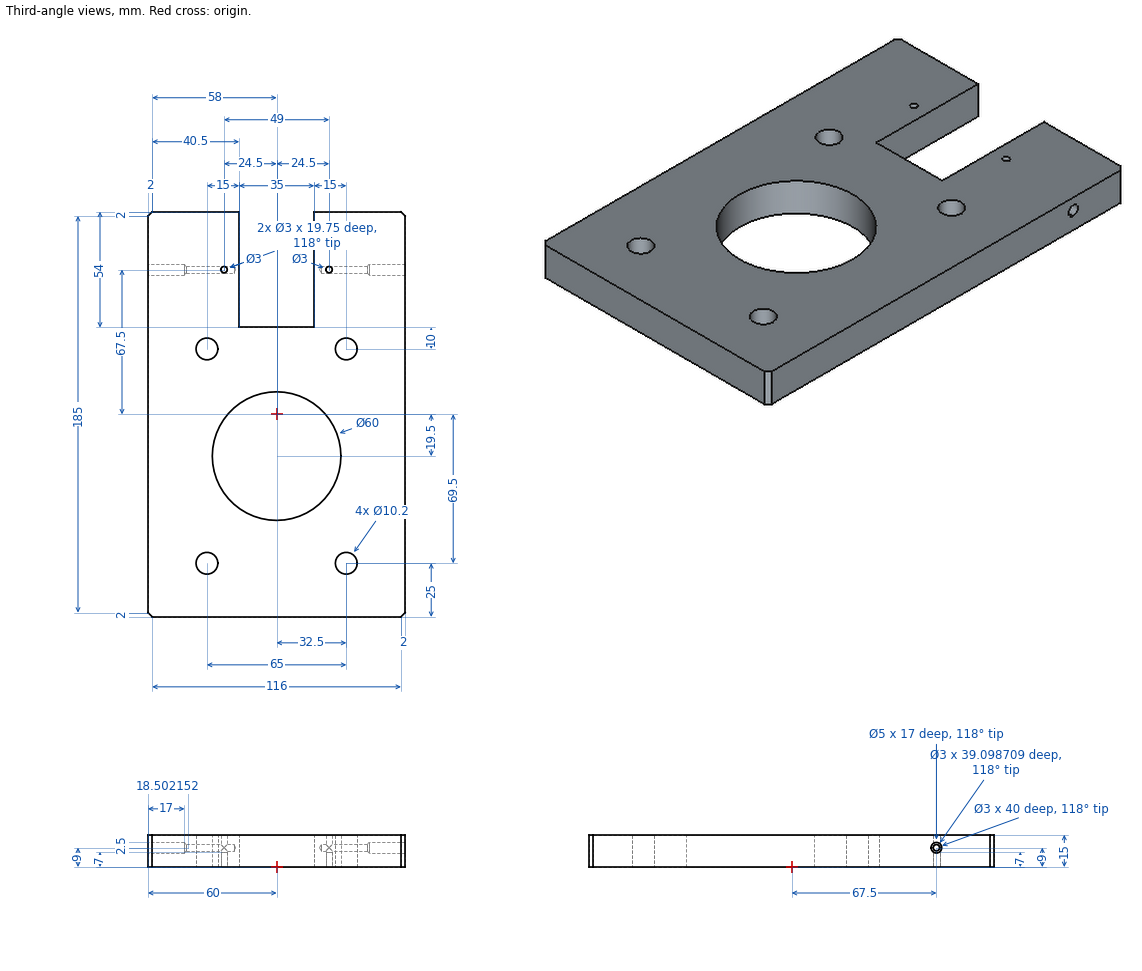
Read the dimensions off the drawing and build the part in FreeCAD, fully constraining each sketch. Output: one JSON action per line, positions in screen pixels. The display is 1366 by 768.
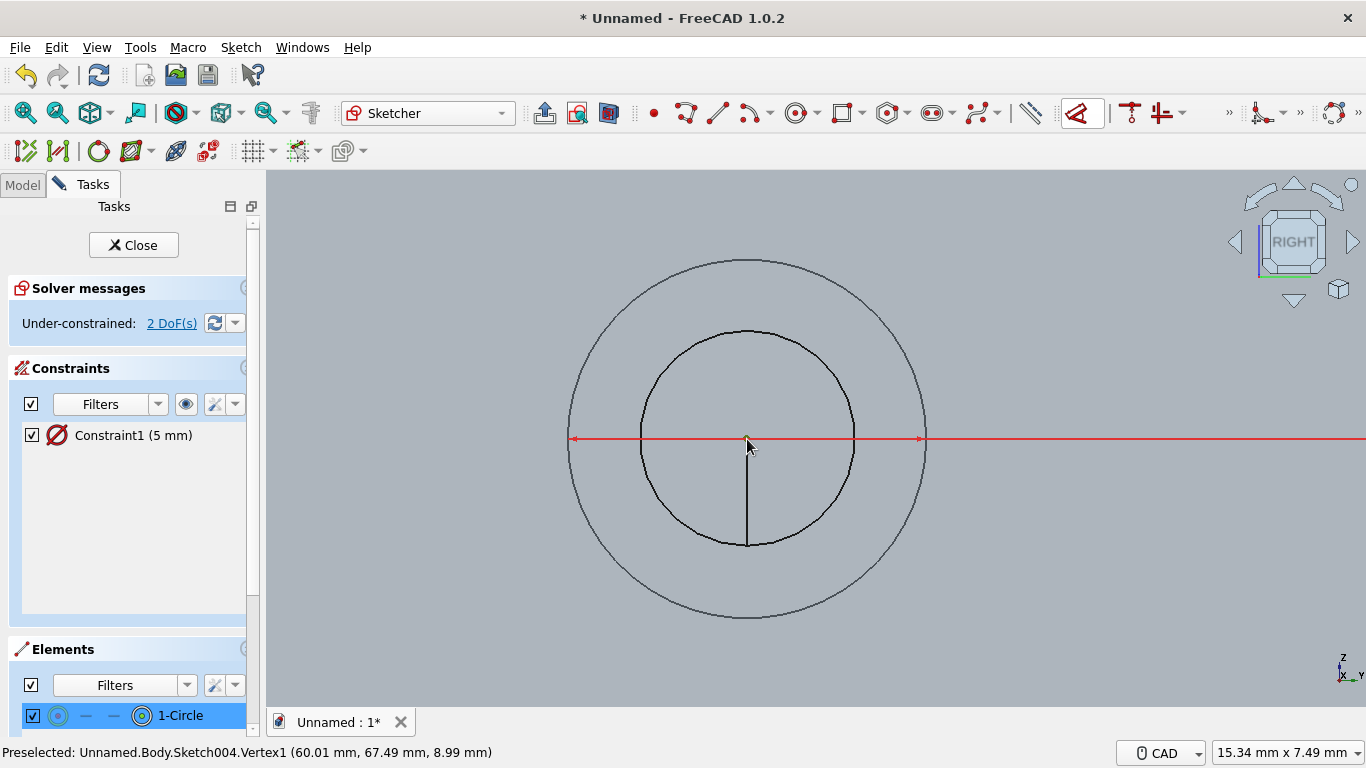
{"action": "key", "text": "i"}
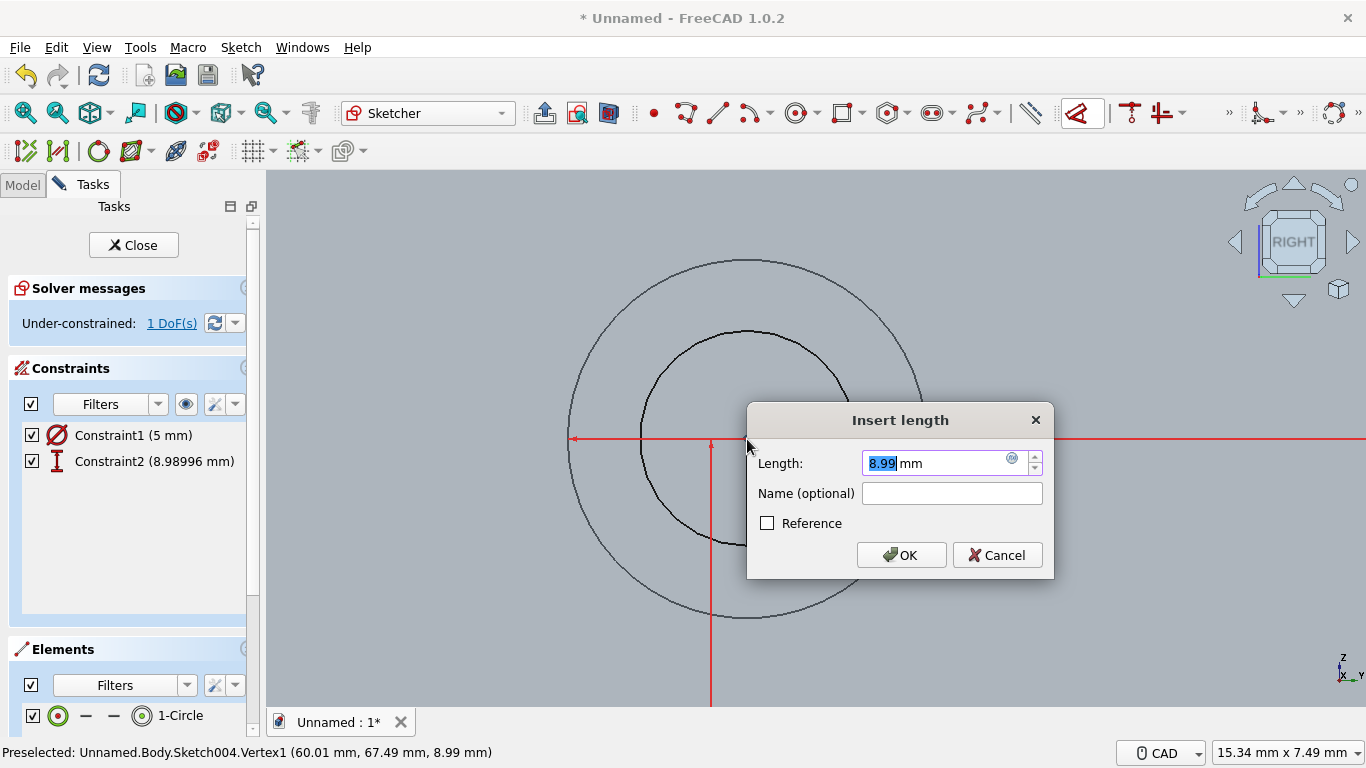
{"action": "type", "text": "9"}
{"action": "key", "text": "Return"}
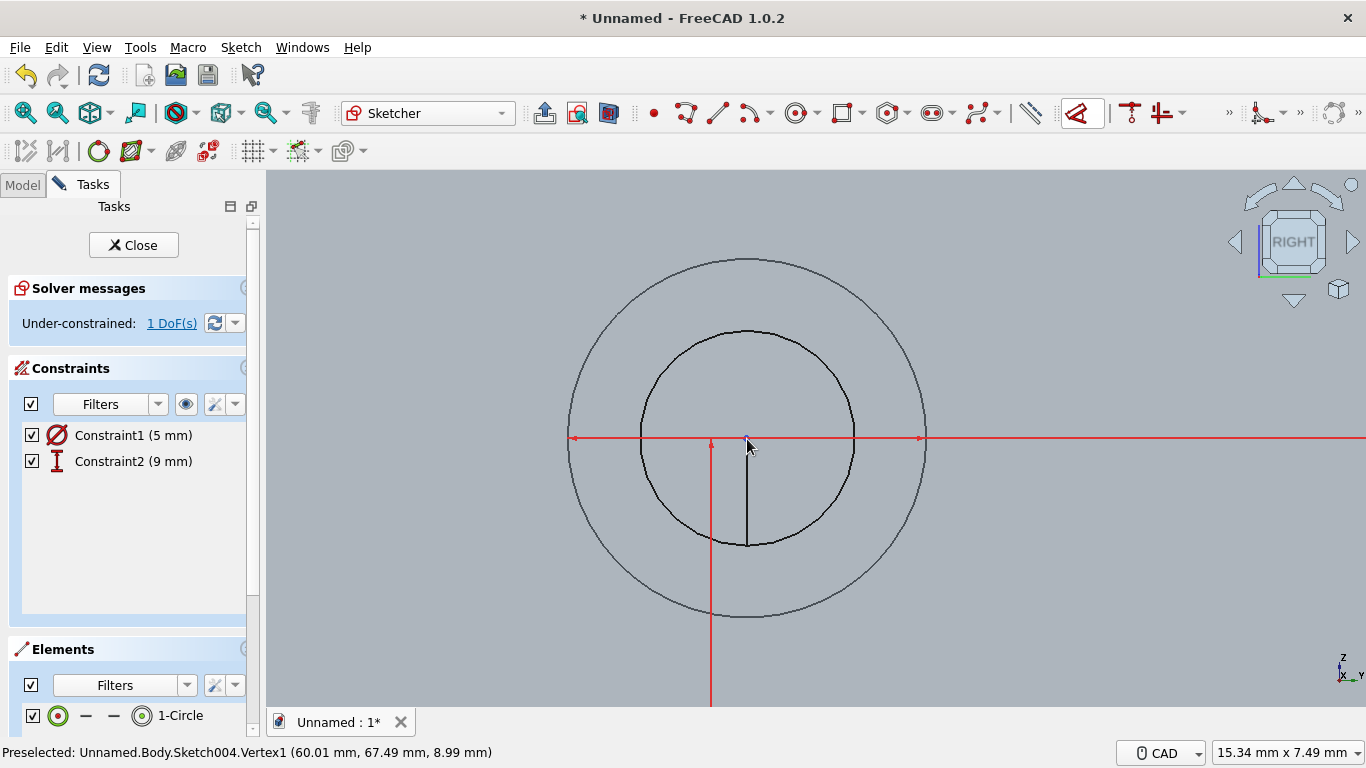
{"action": "left_click", "coordinate": [747, 438]}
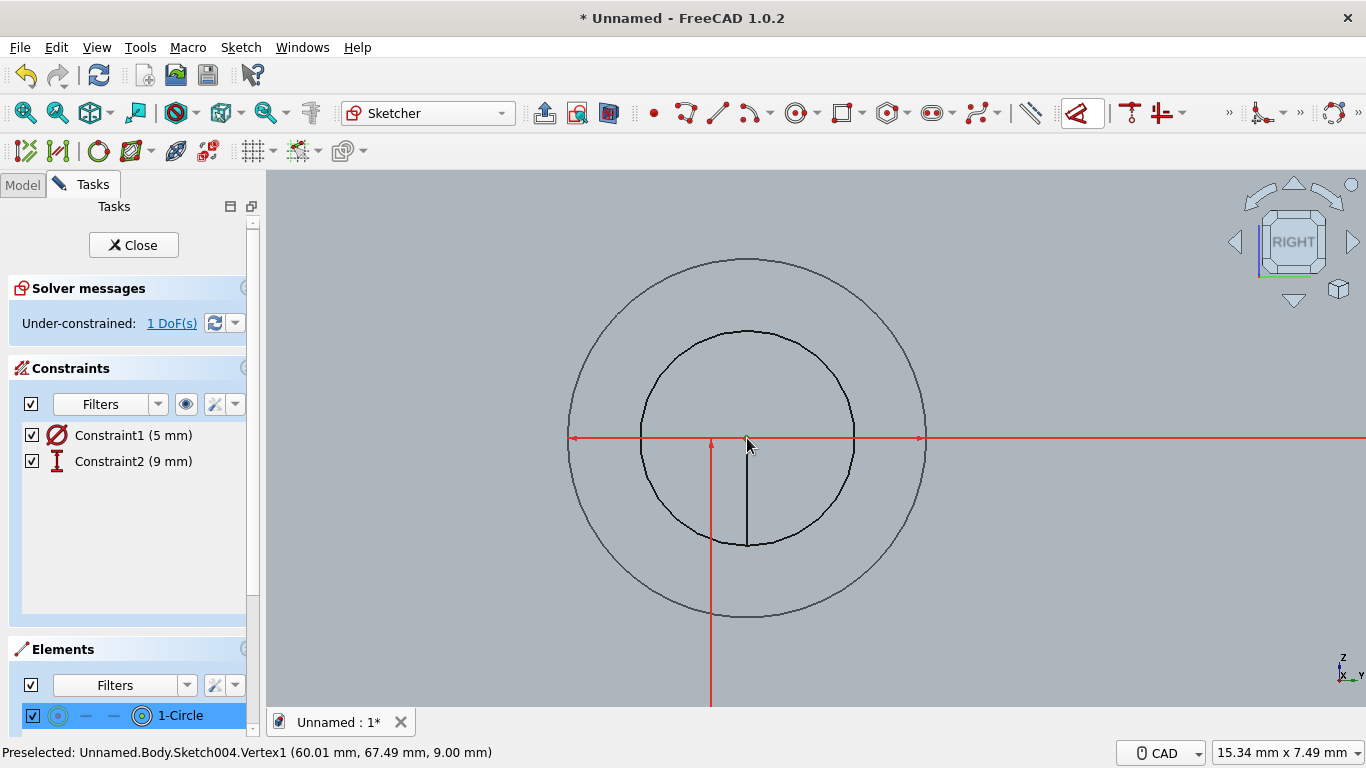
{"action": "key", "text": "l"}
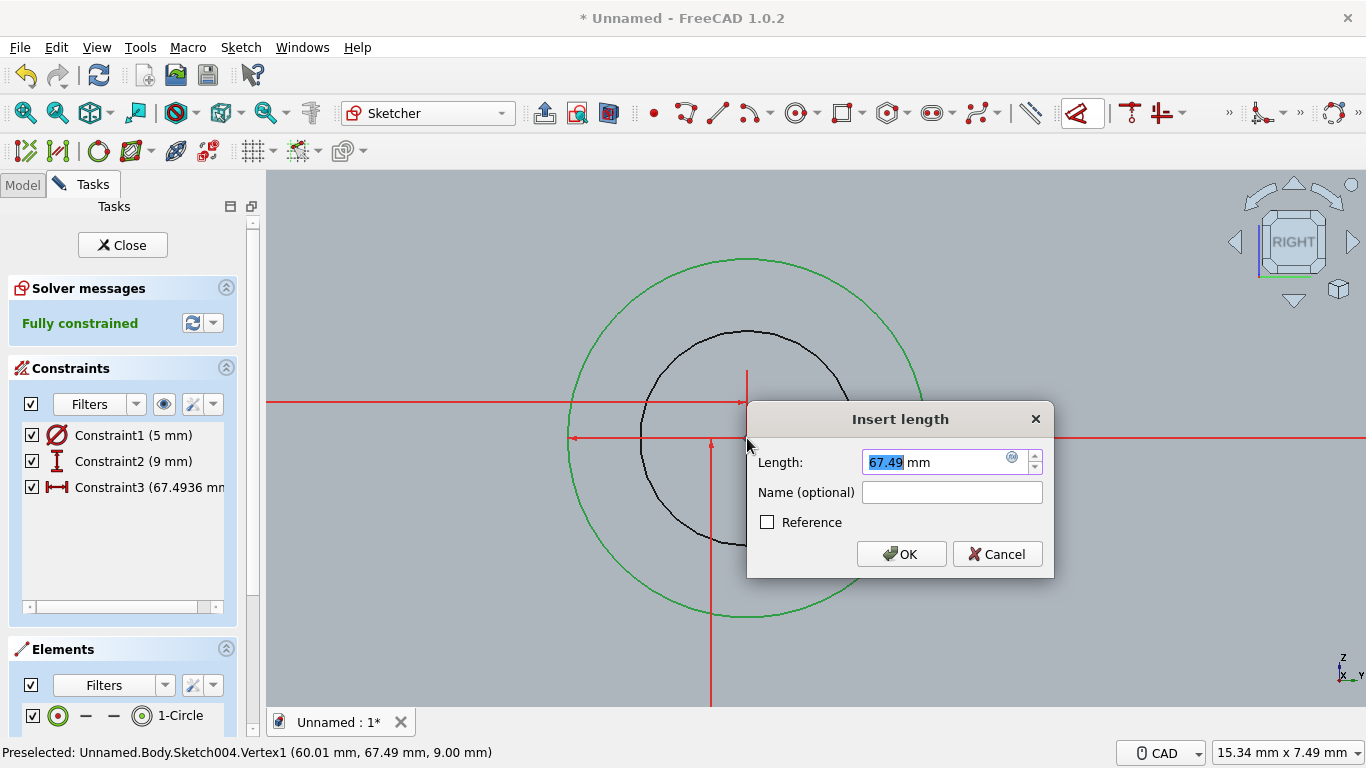
{"action": "type", "text": "67.5"}
{"action": "key", "text": "Return"}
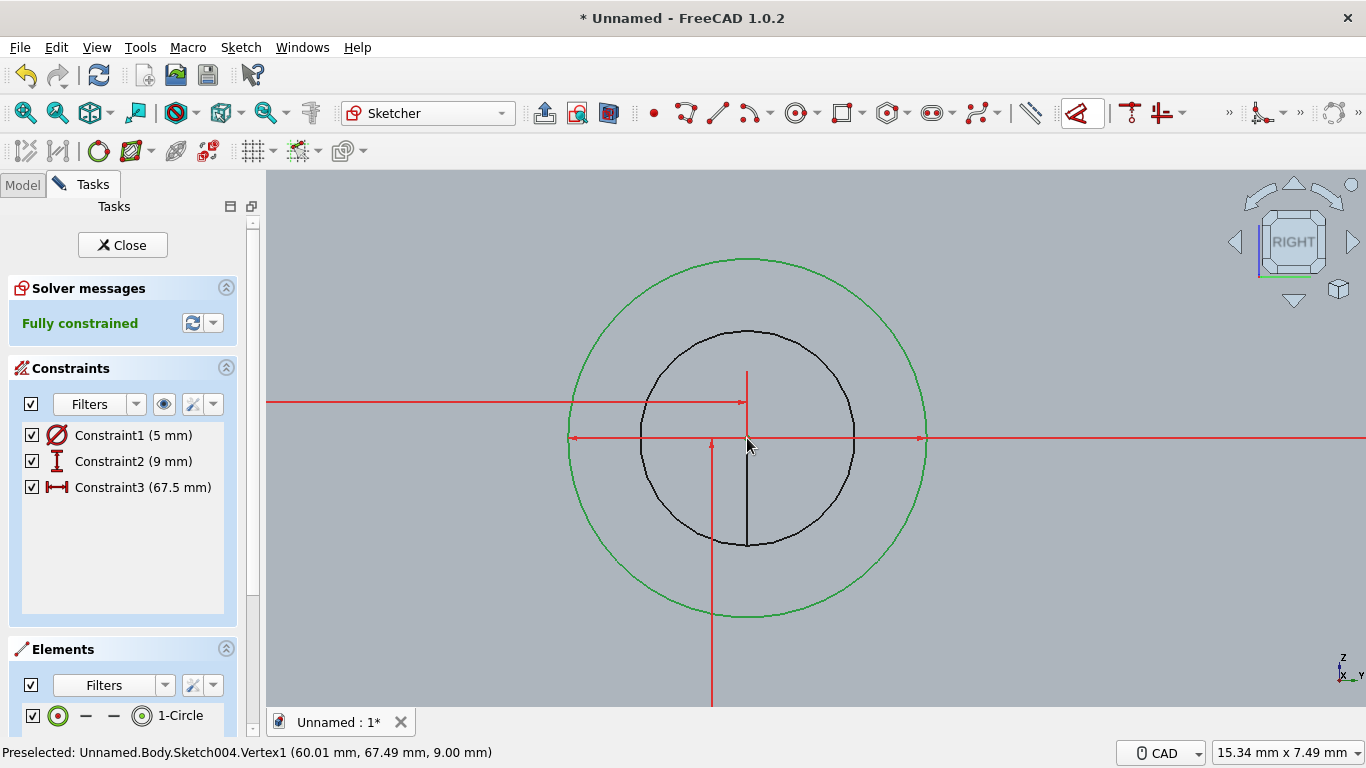
{"action": "left_click", "coordinate": [123, 245]}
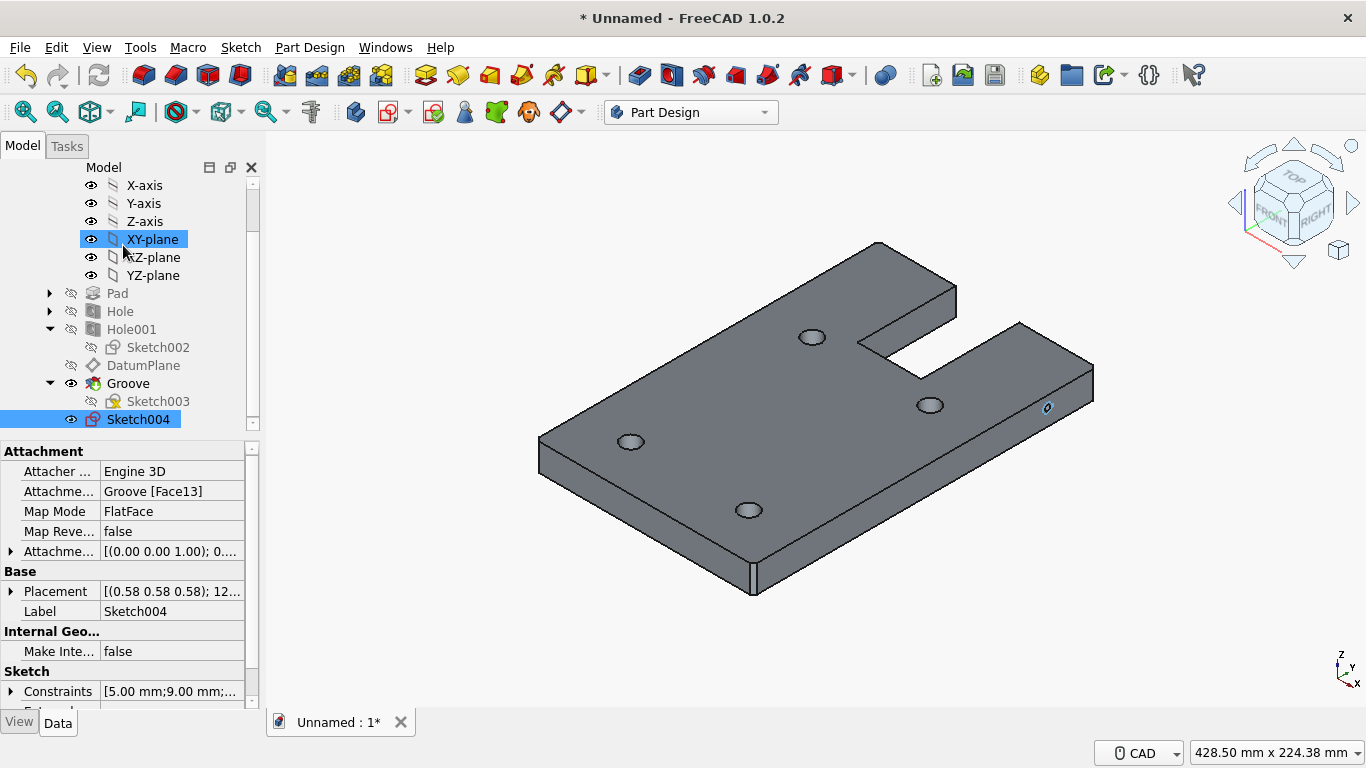
{"action": "left_click", "coordinate": [672, 76]}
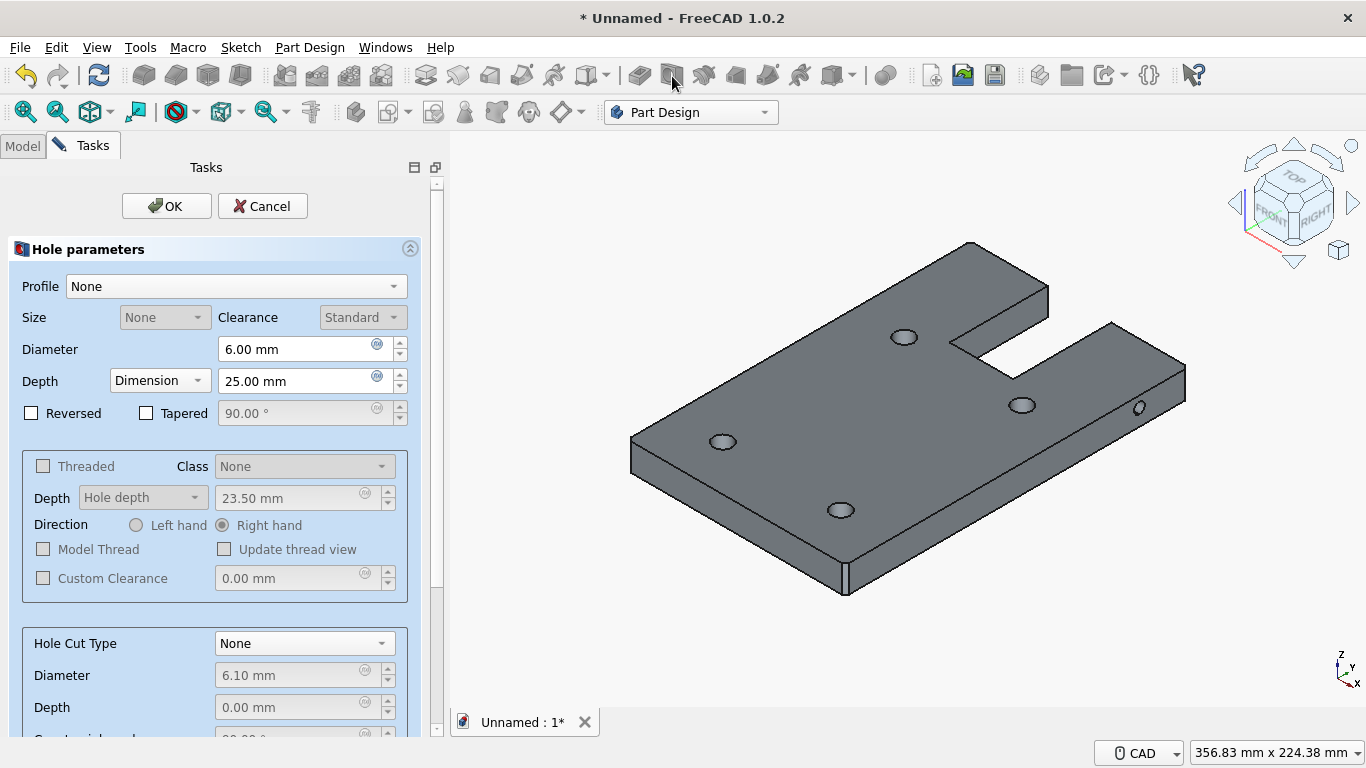
{"action": "triple_click", "coordinate": [305, 349]}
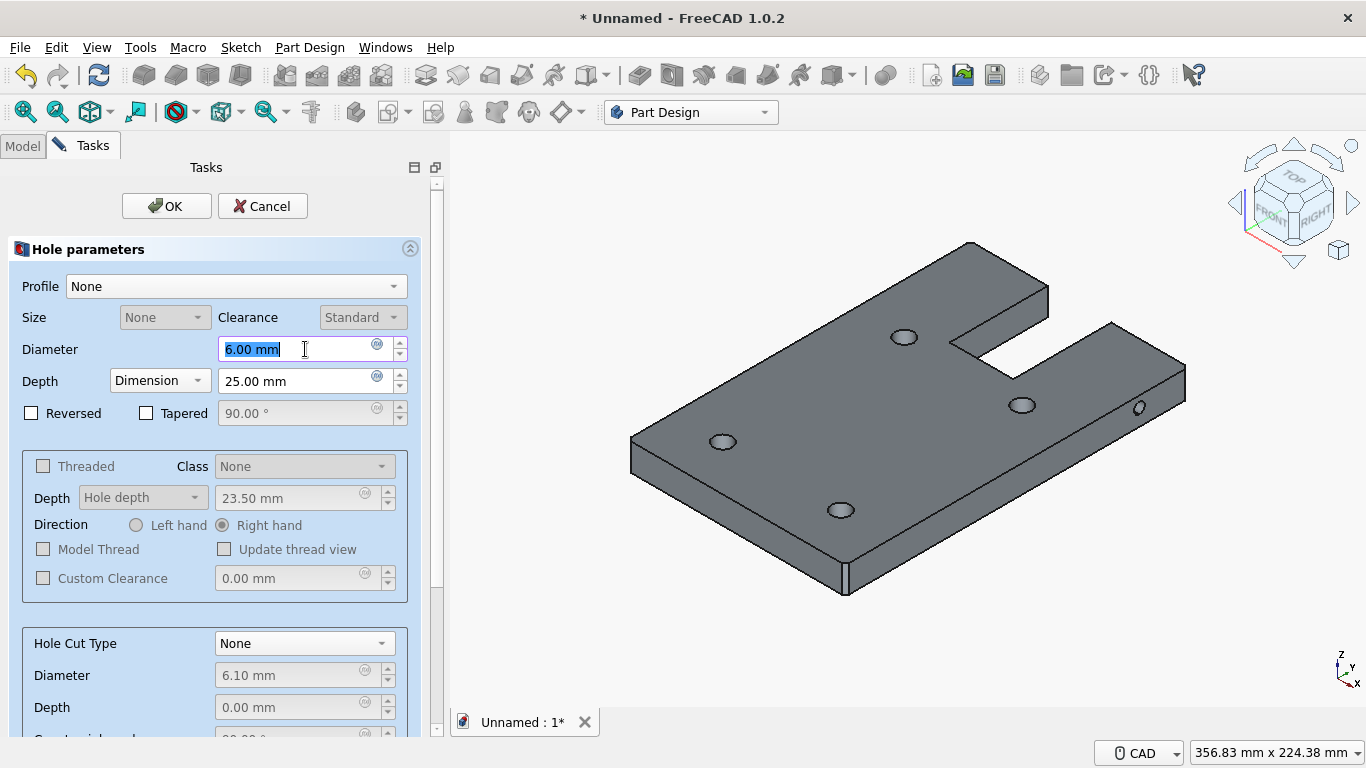
{"action": "type", "text": "5"}
{"action": "key", "text": "Tab"}